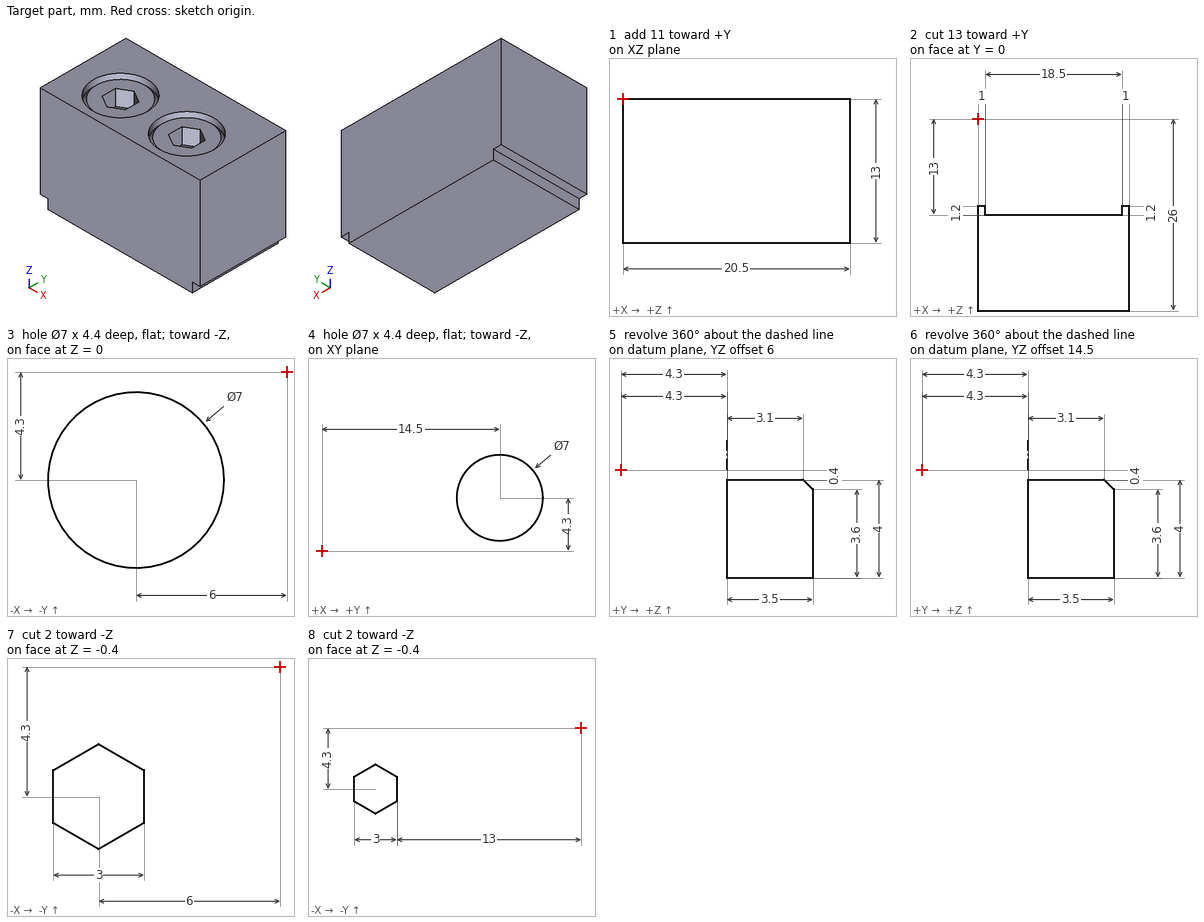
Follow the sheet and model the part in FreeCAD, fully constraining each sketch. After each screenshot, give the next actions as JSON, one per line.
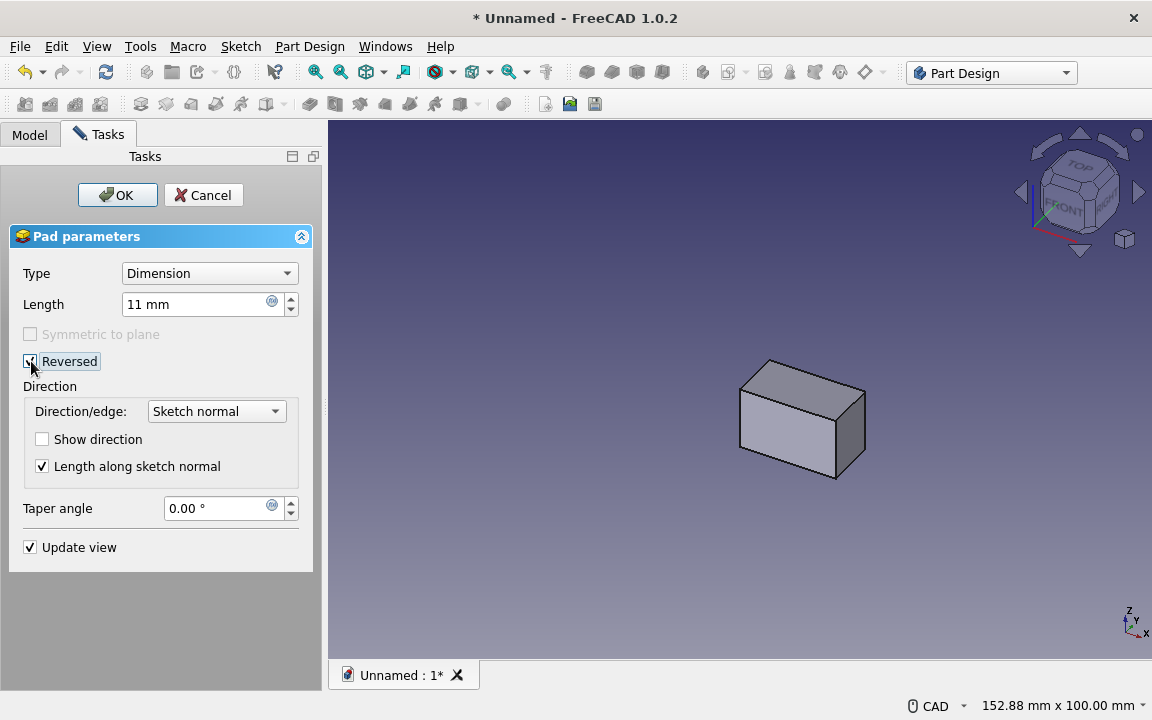
{"action": "left_click", "coordinate": [118, 195]}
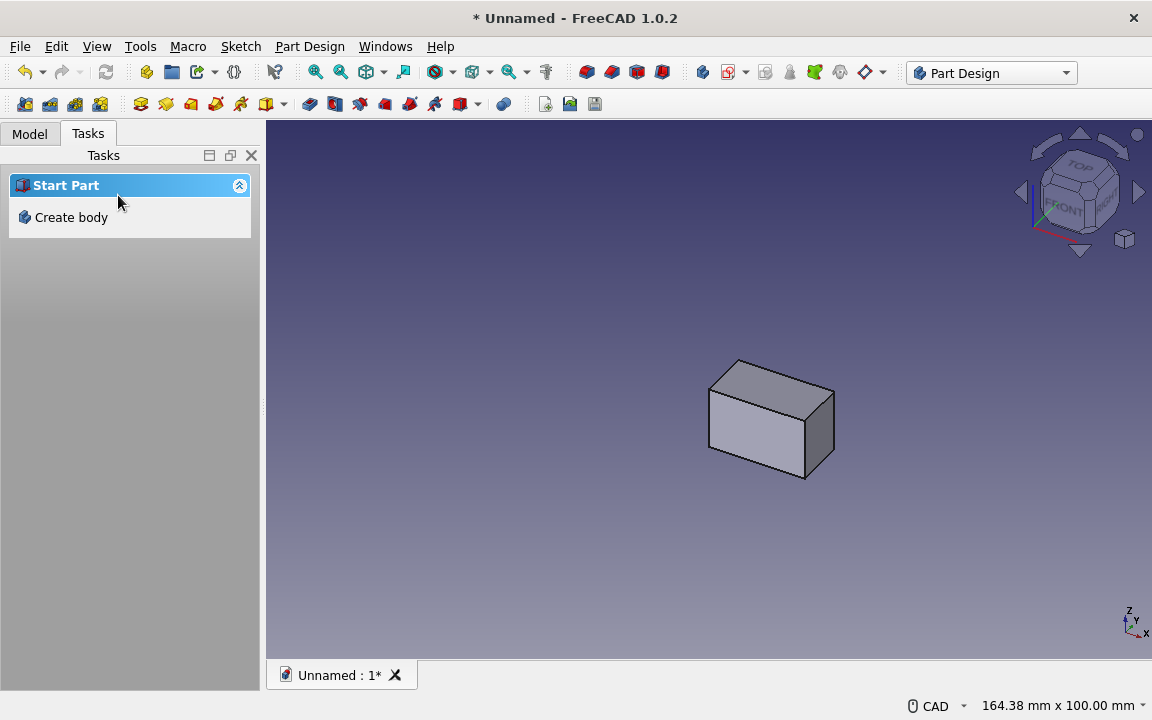
{"action": "left_click", "coordinate": [316, 72]}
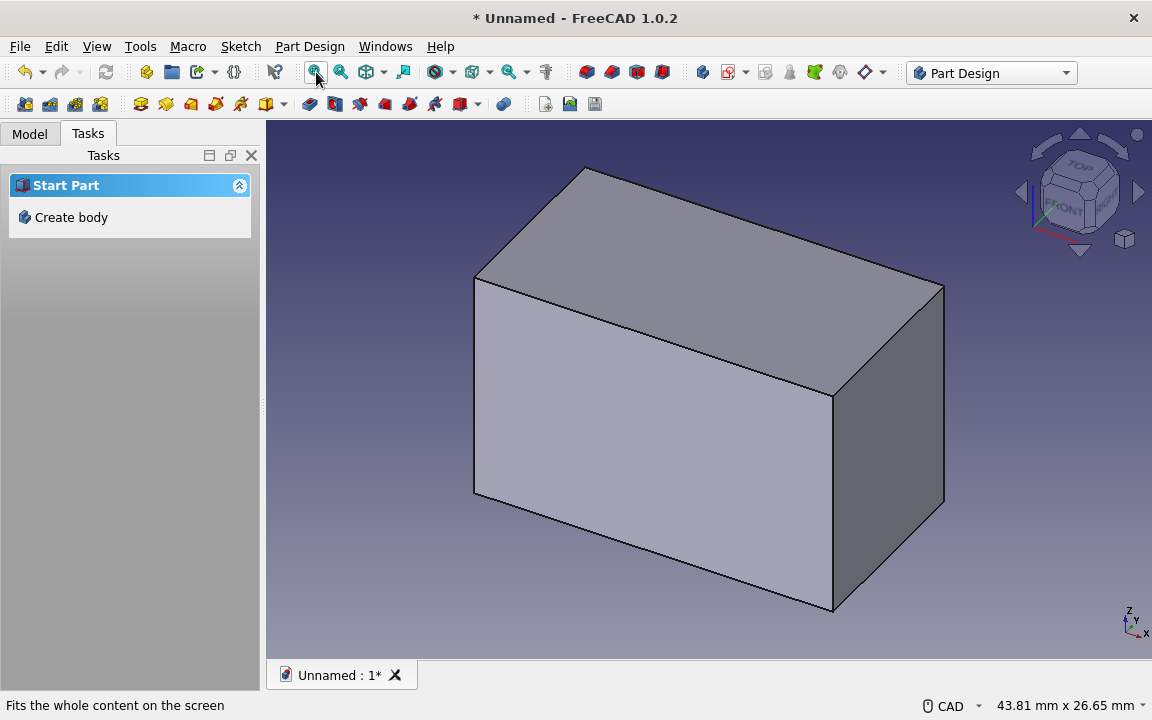
{"action": "left_click", "coordinate": [705, 461]}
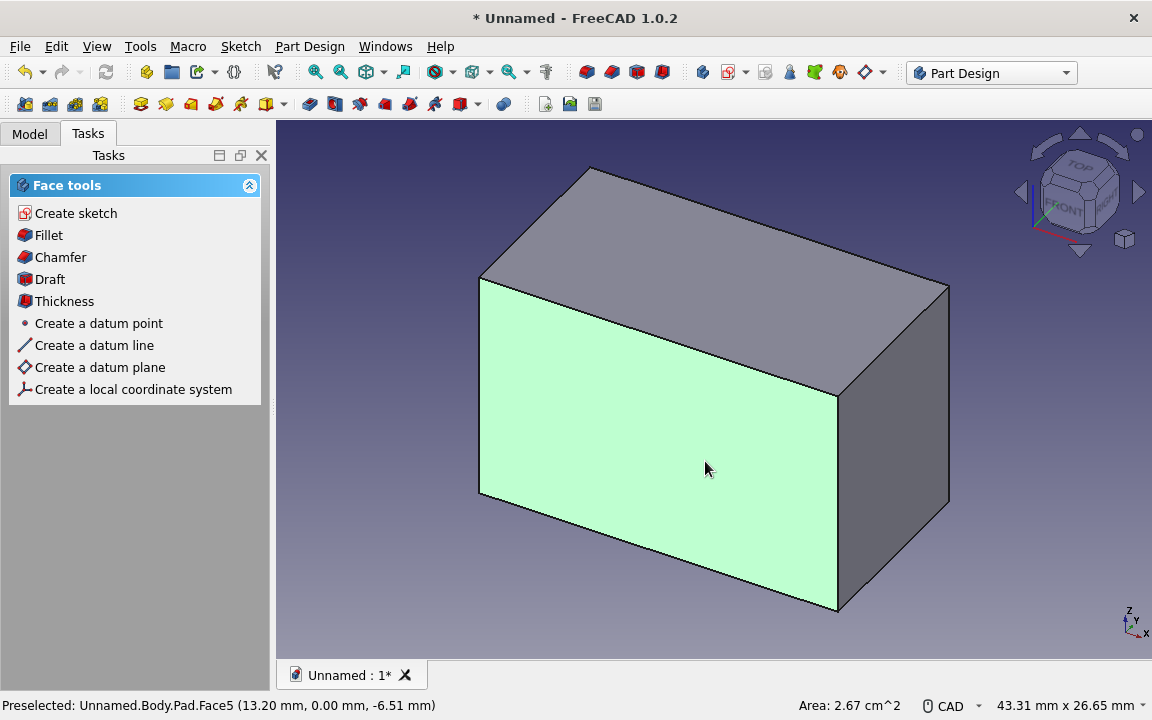
{"action": "left_click", "coordinate": [728, 72]}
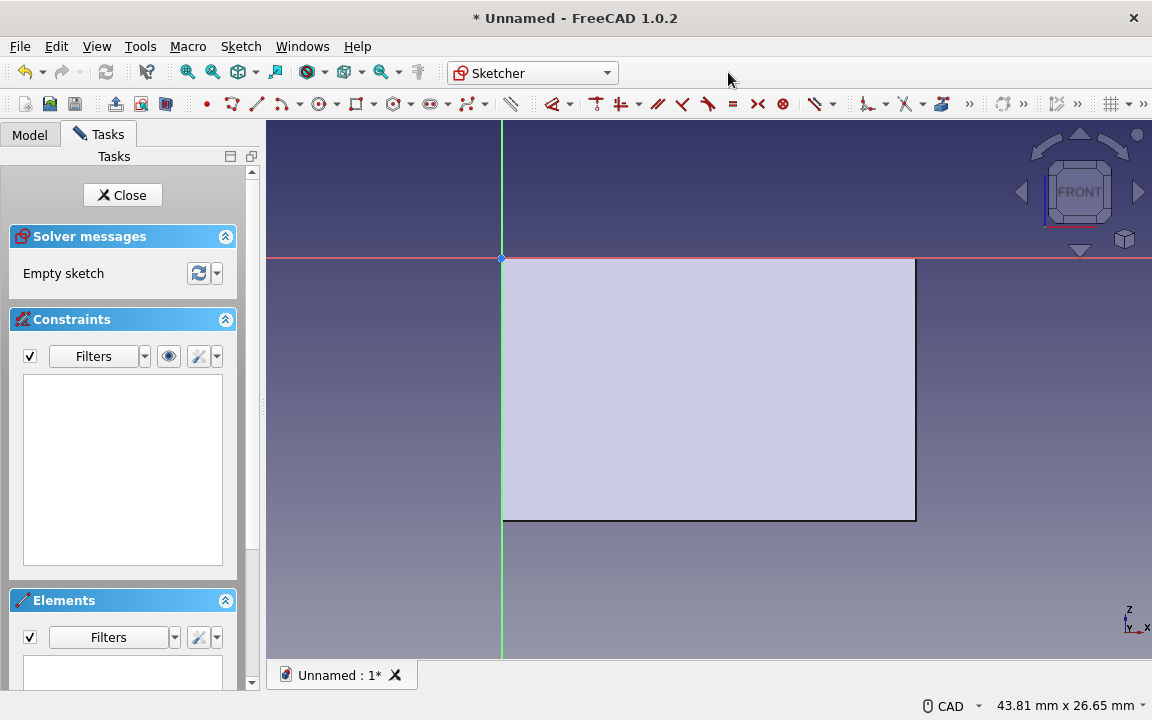
{"action": "scroll", "coordinate": [501, 148], "scroll_direction": "down", "scroll_amount": 2}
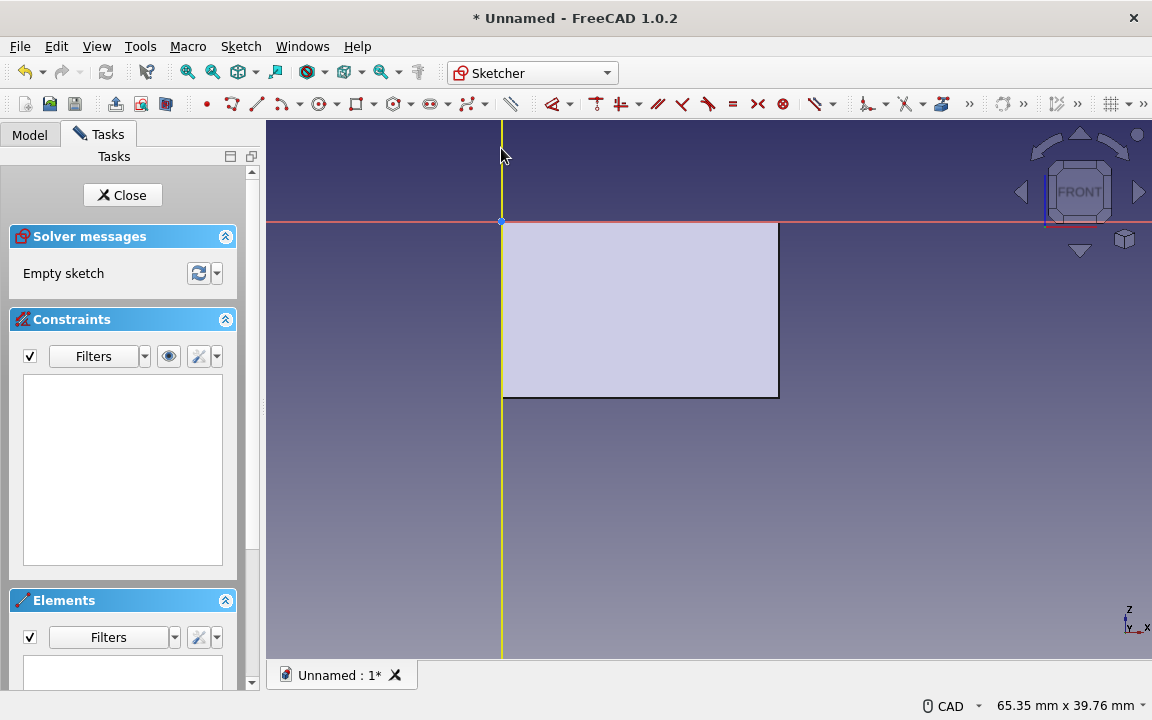
{"action": "left_click", "coordinate": [232, 104]}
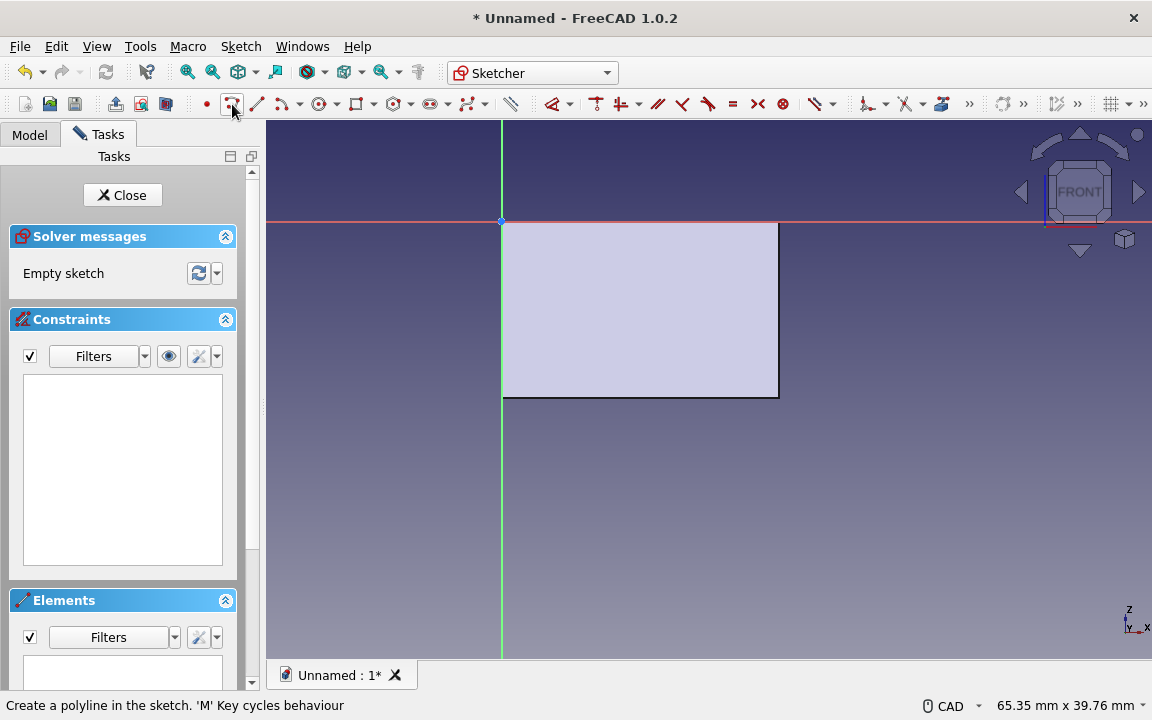
{"action": "left_click", "coordinate": [502, 382]}
{"action": "left_click", "coordinate": [515, 382]}
{"action": "left_click", "coordinate": [515, 398]}
{"action": "left_click", "coordinate": [766, 398]}
{"action": "left_click", "coordinate": [766, 382]}
{"action": "left_click", "coordinate": [779, 382]}
{"action": "left_click", "coordinate": [779, 574]}
{"action": "left_click", "coordinate": [511, 574]}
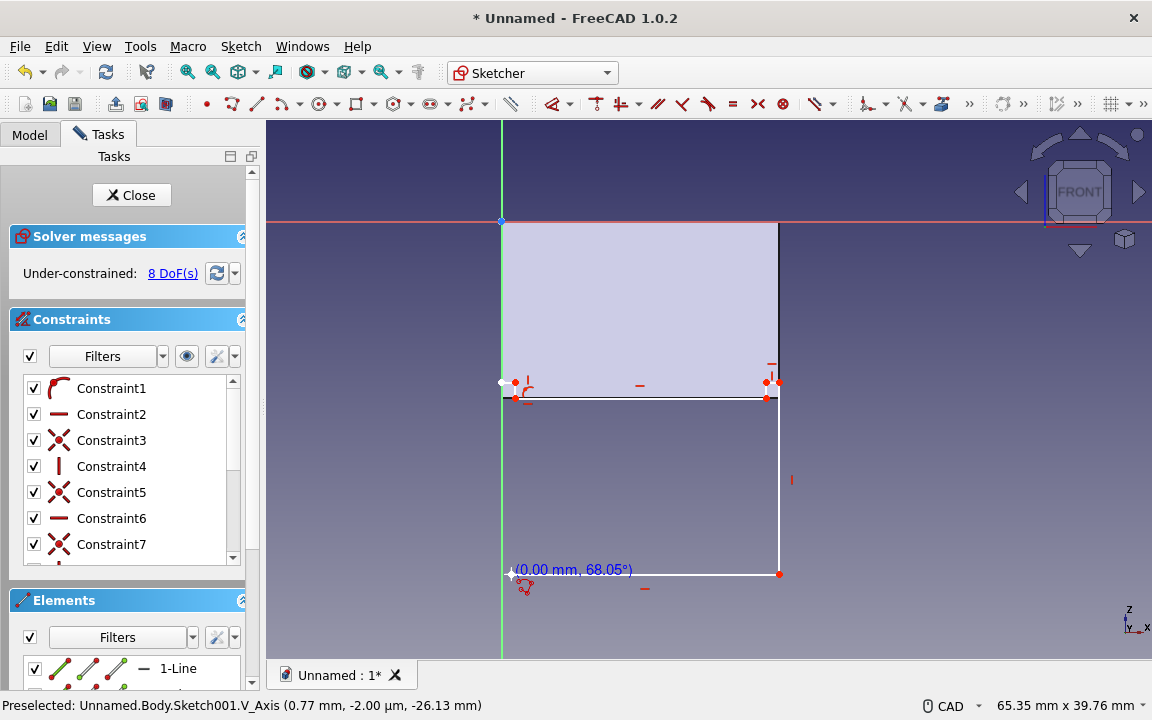
{"action": "scroll", "coordinate": [502, 382], "scroll_direction": "up", "scroll_amount": 5}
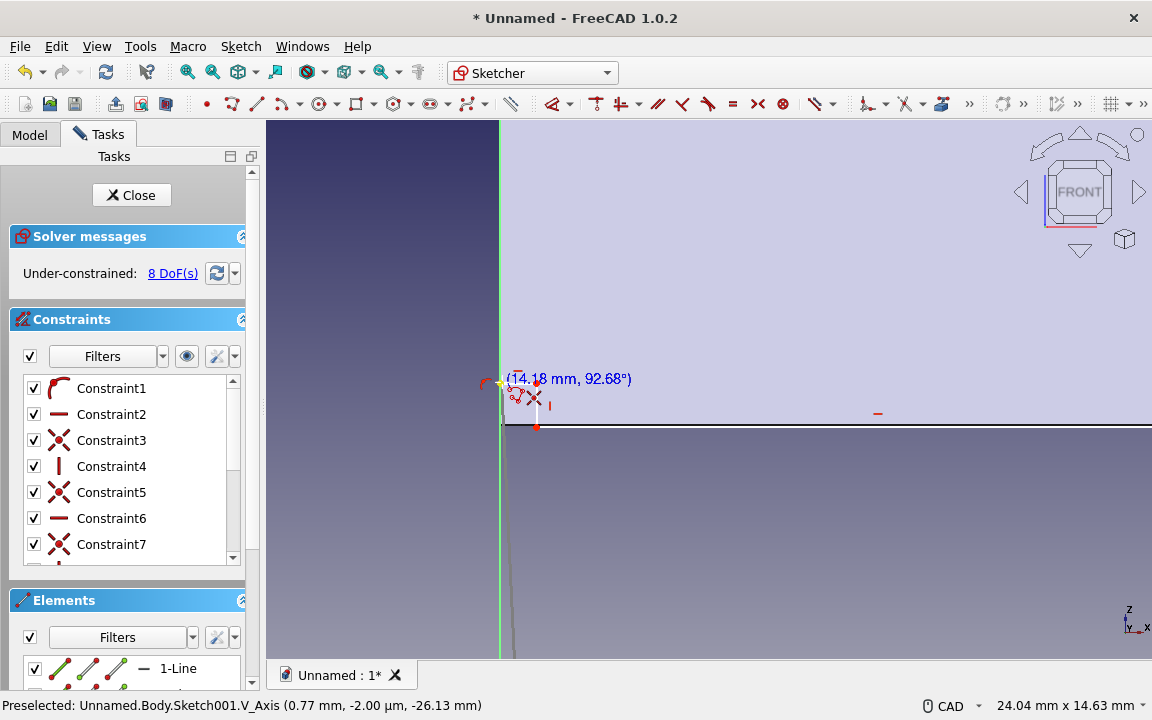
{"action": "left_click", "coordinate": [500, 384]}
{"action": "key", "text": "Escape"}
{"action": "key", "text": "Escape"}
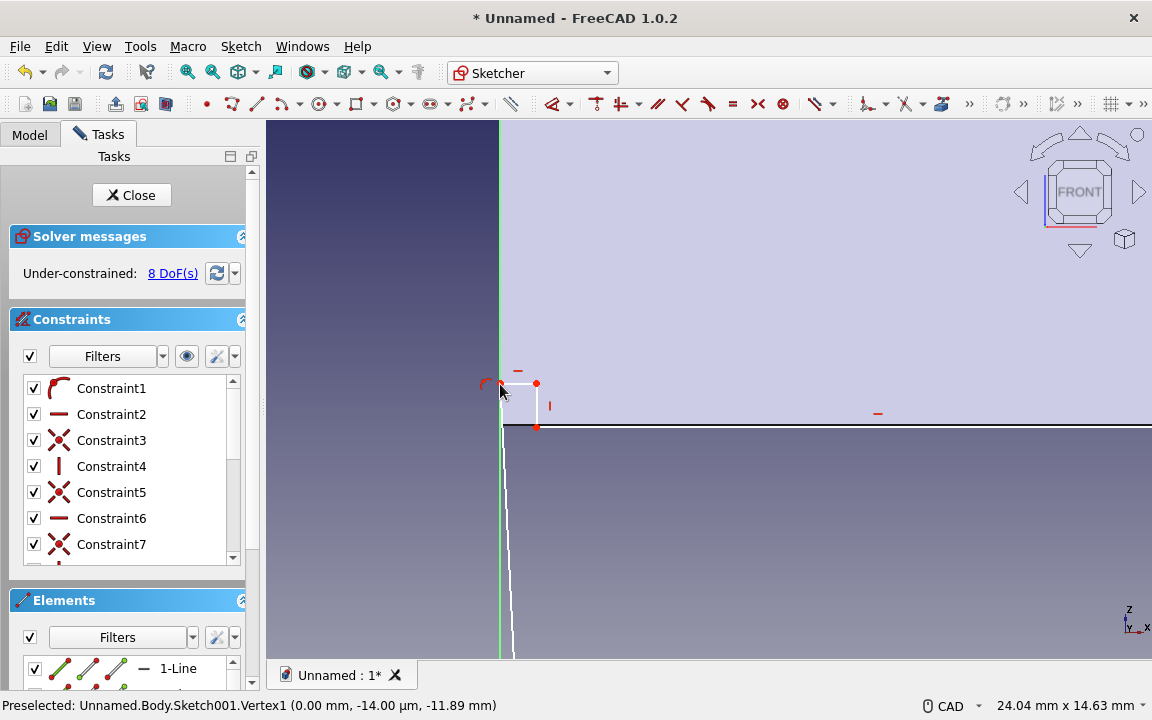
{"action": "scroll", "coordinate": [511, 593], "scroll_direction": "up", "scroll_amount": 2}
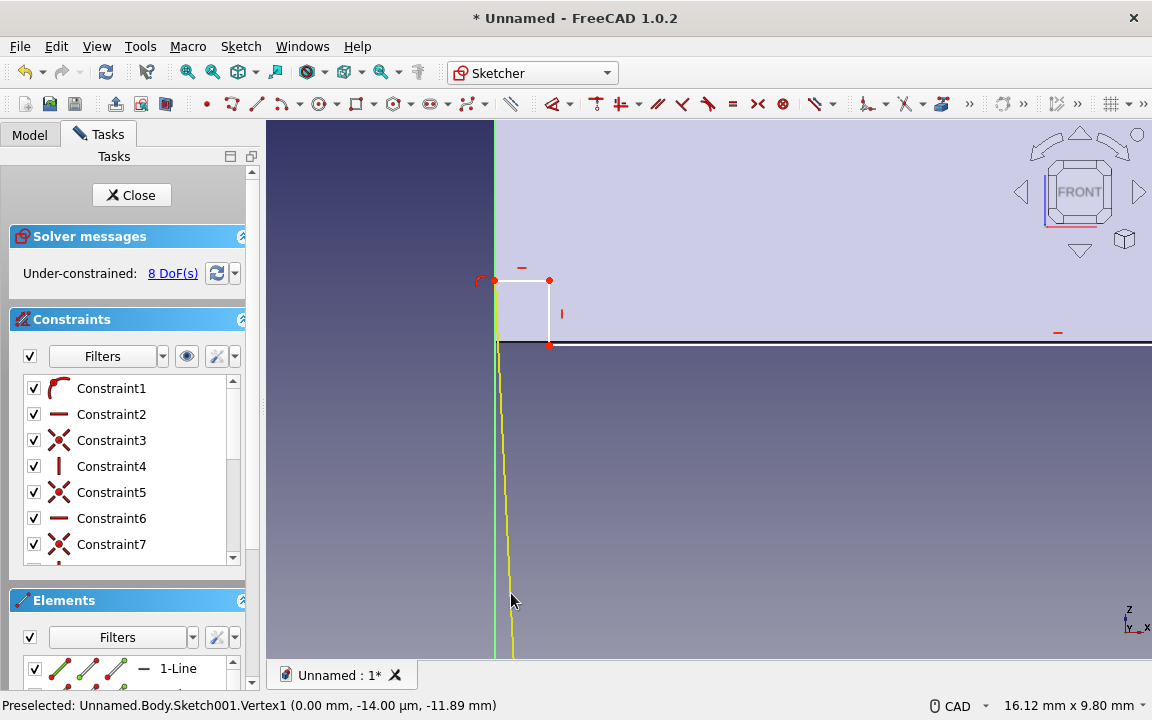
{"action": "left_click", "coordinate": [510, 592]}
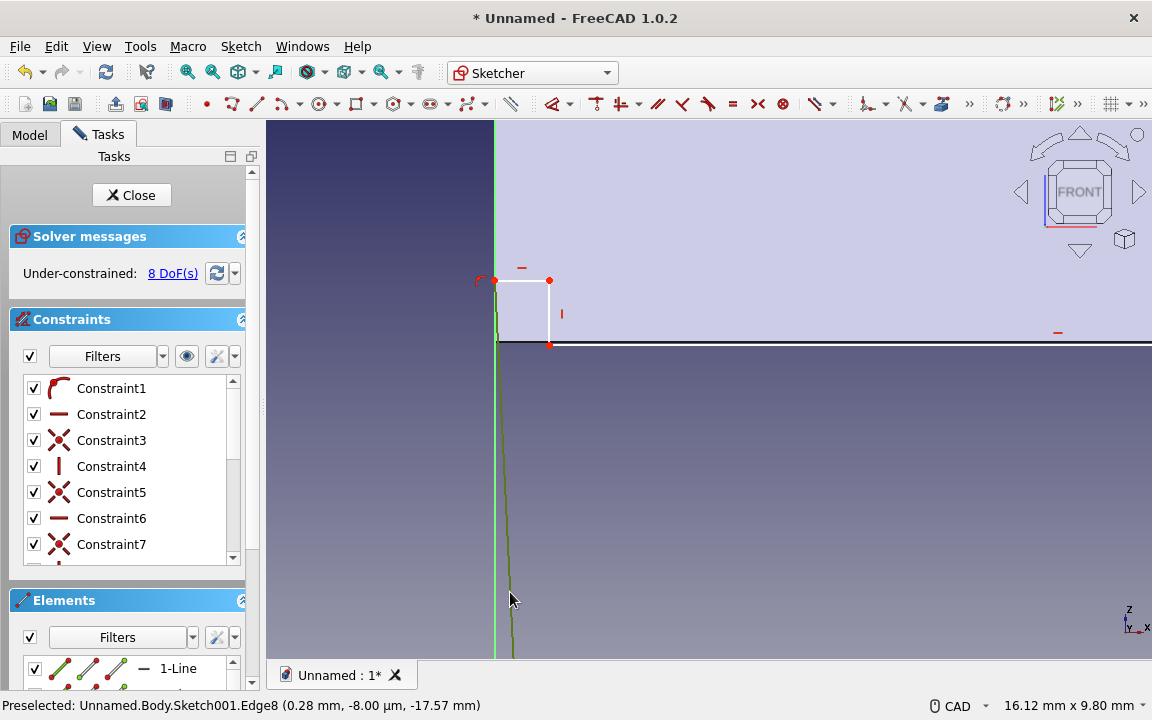
{"action": "key", "text": "v"}